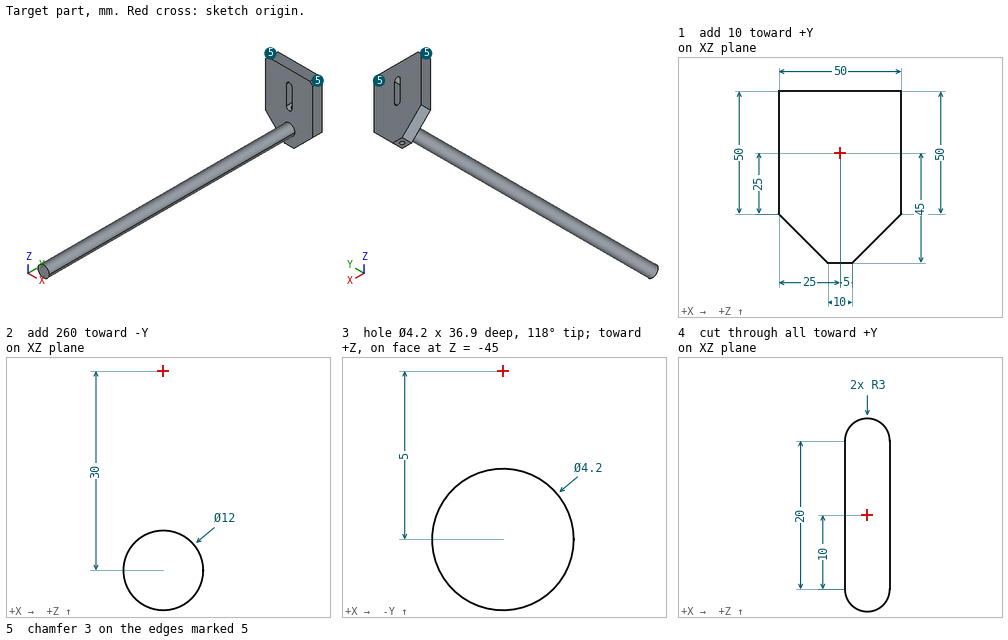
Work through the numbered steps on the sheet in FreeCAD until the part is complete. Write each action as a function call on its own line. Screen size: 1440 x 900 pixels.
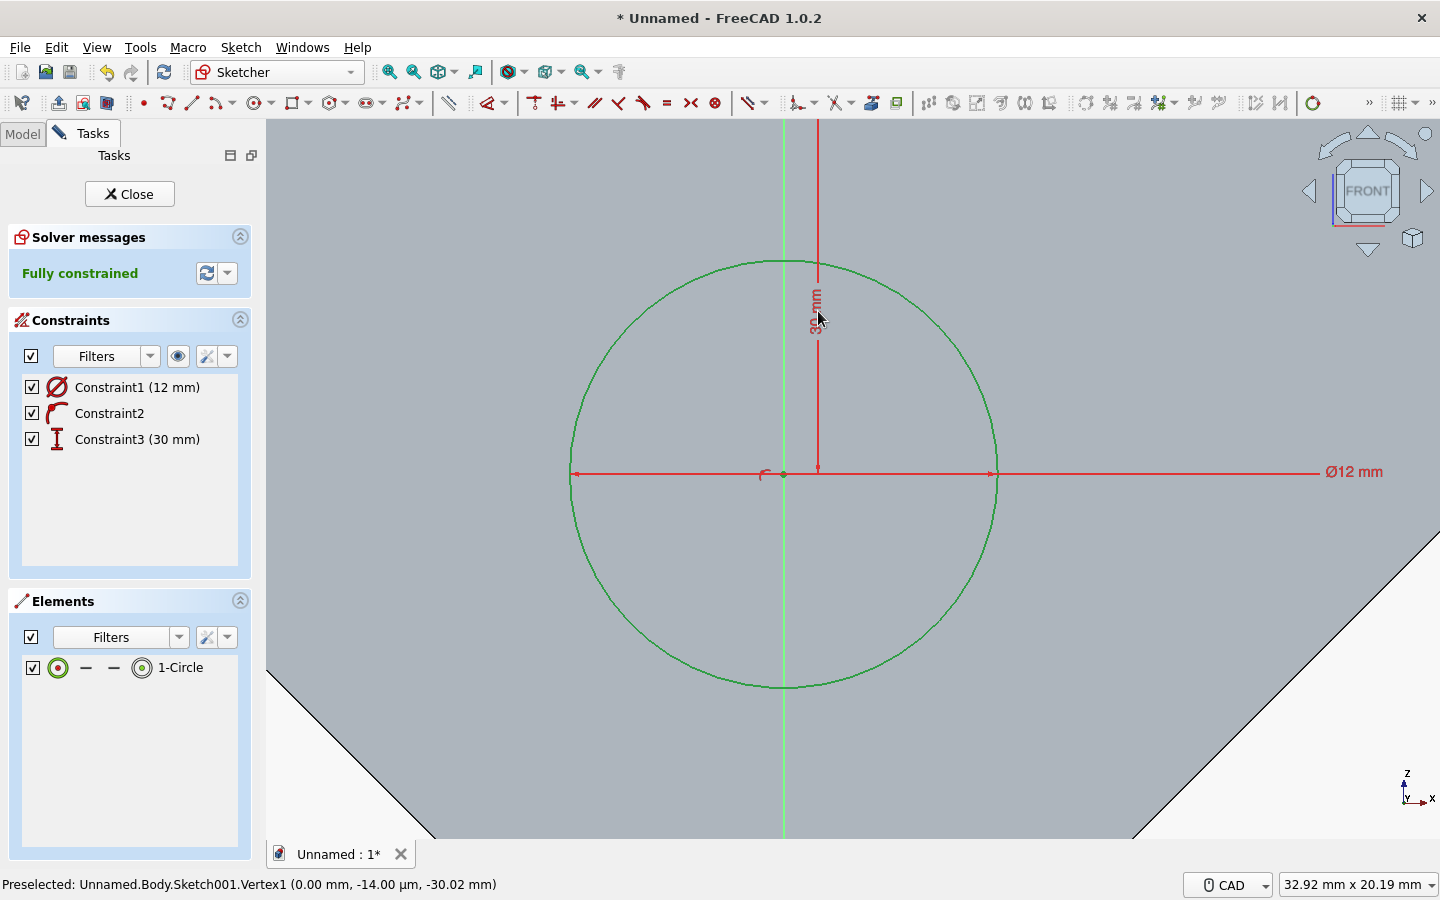
click(130, 194)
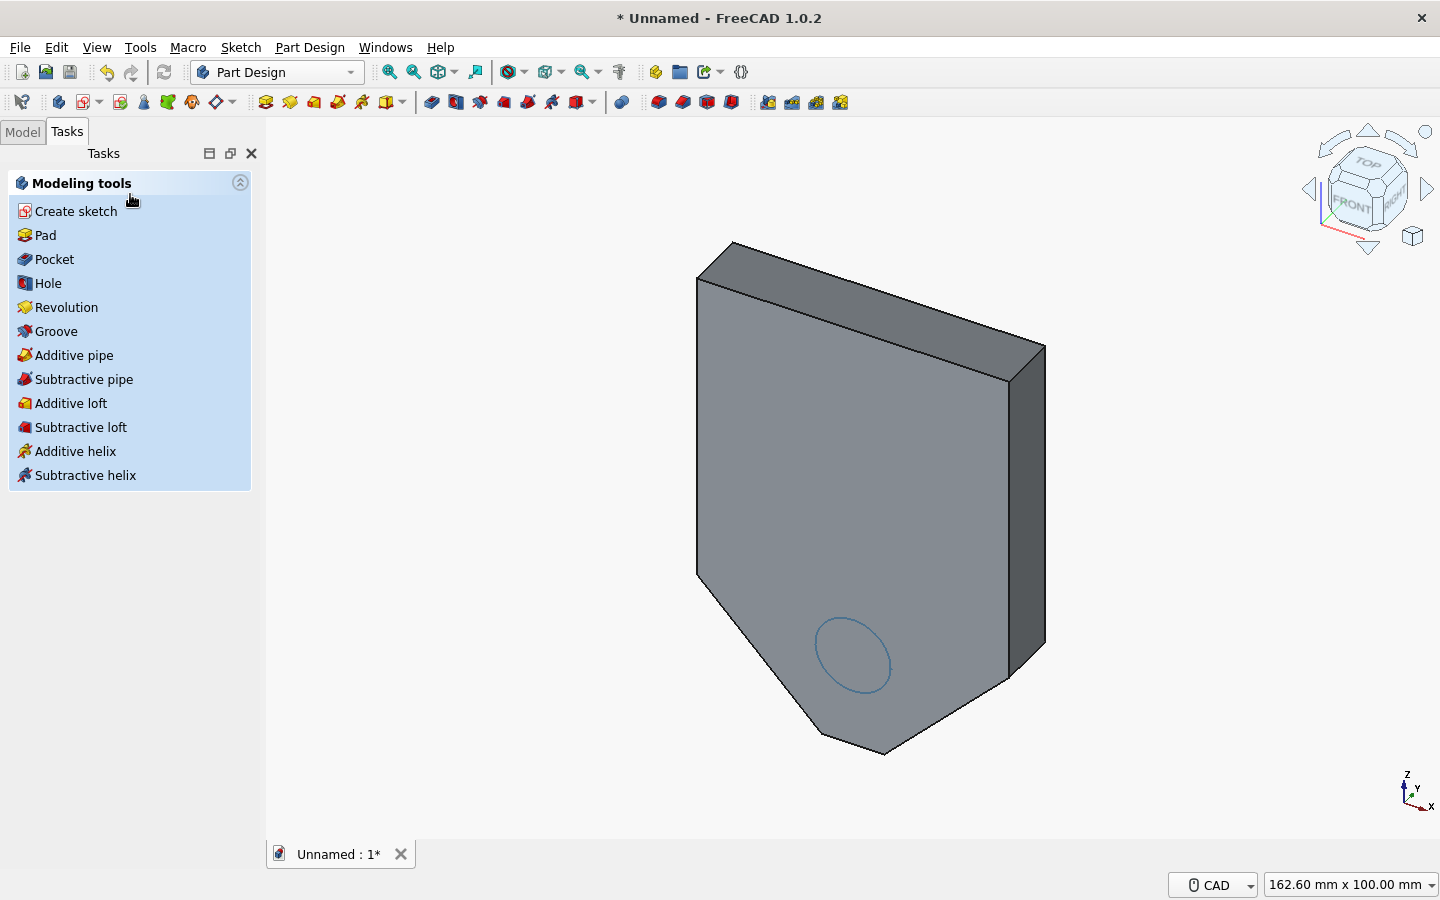
click(266, 102)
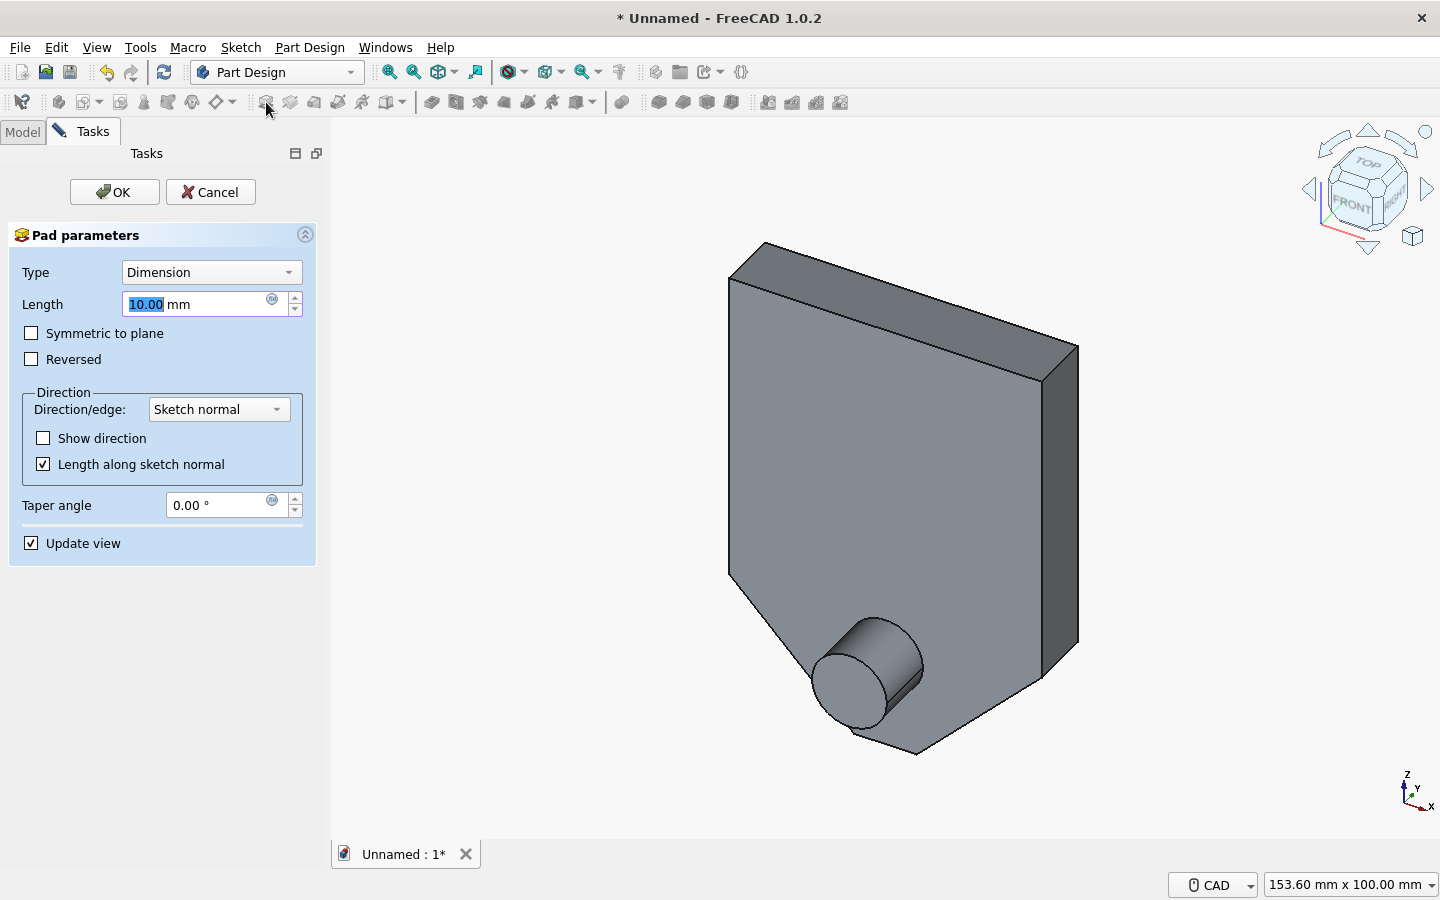
text(260)
key(Tab)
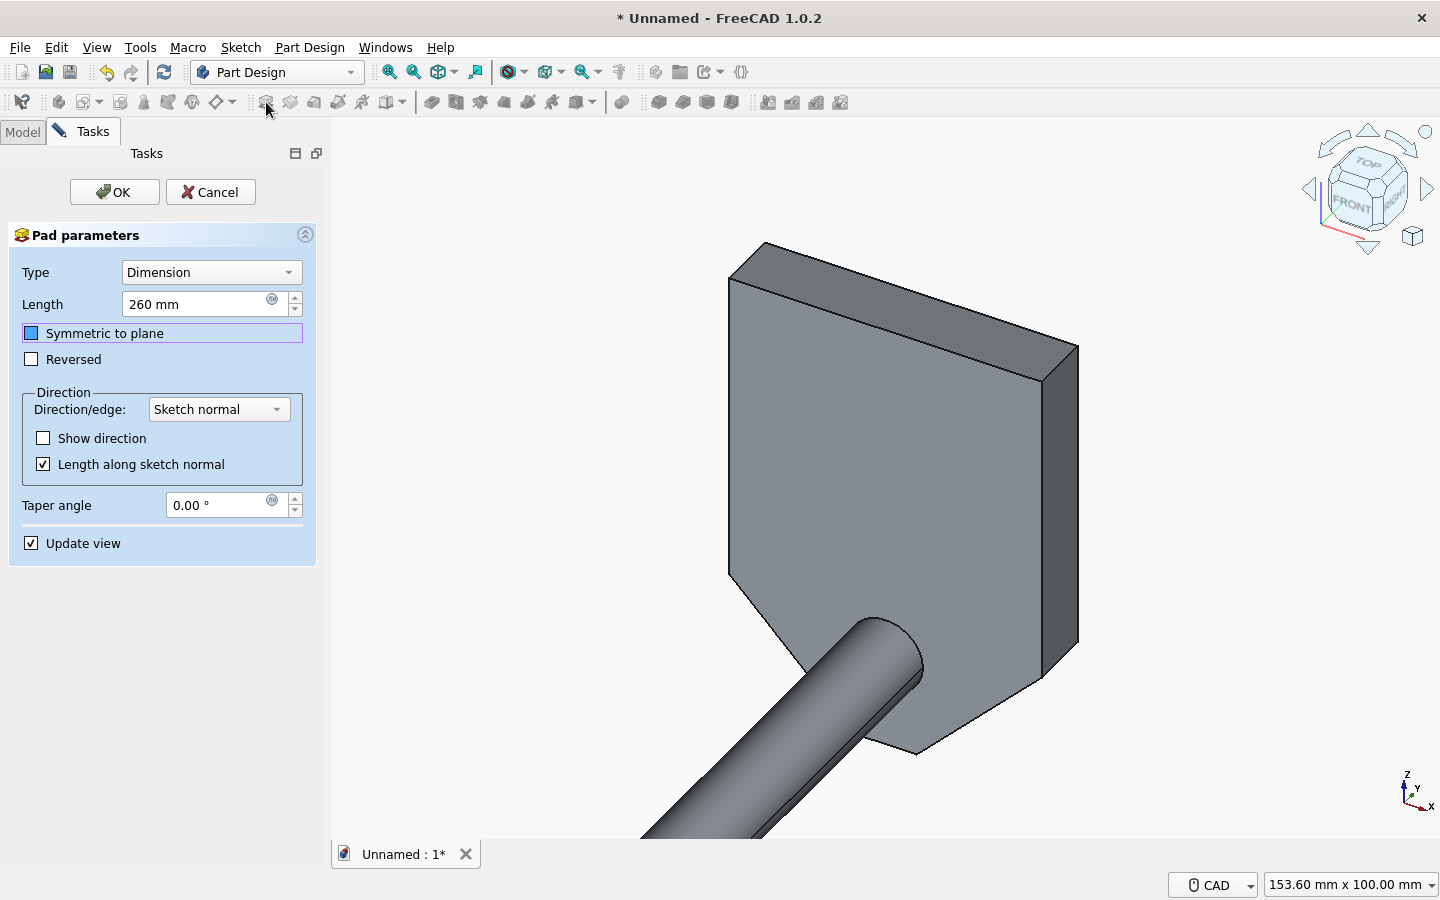
click(115, 192)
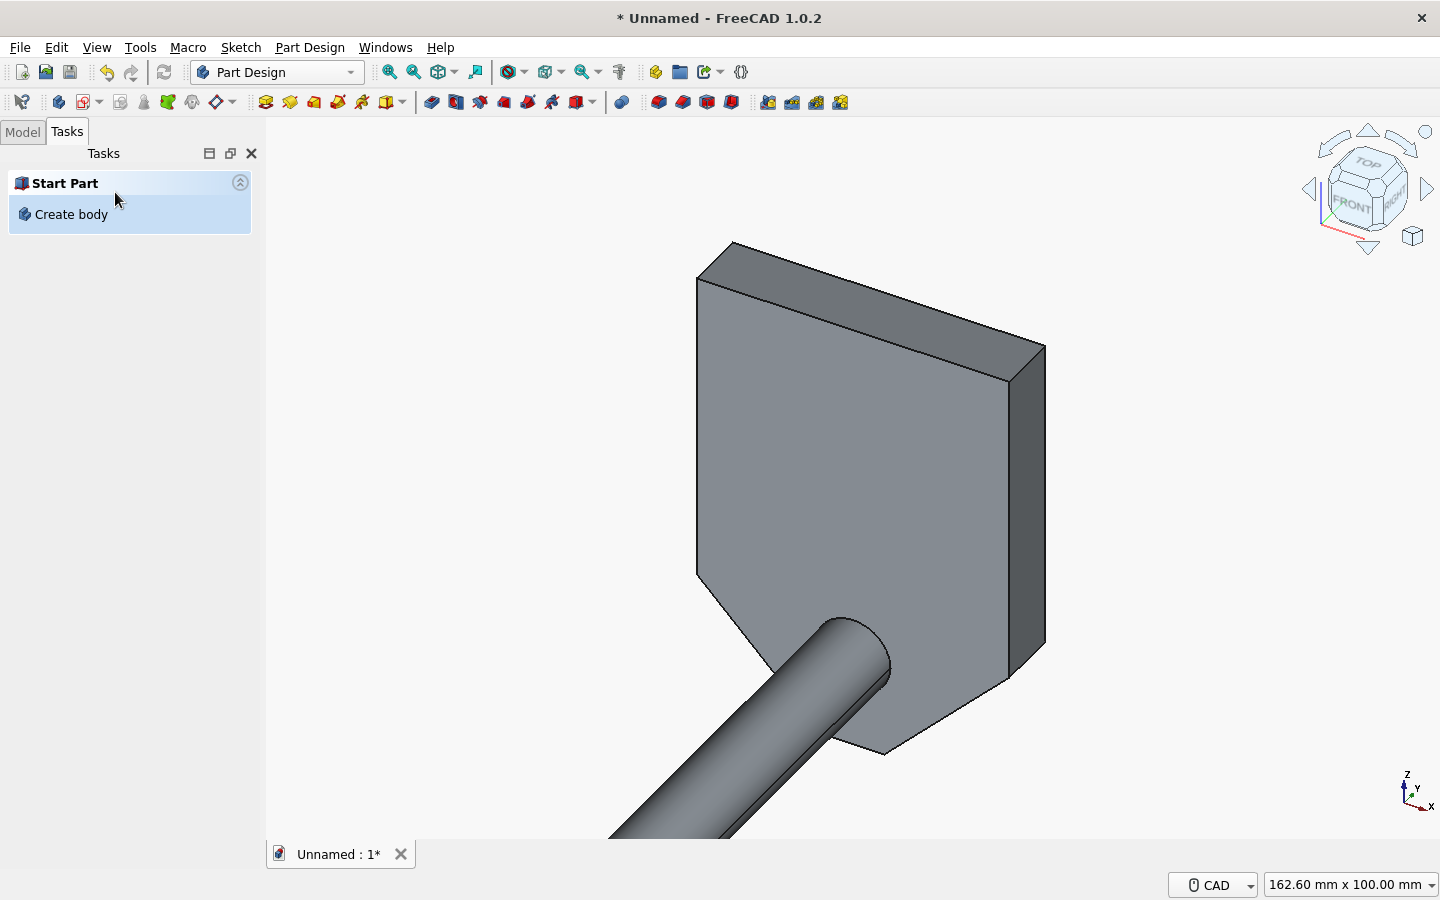
click(390, 72)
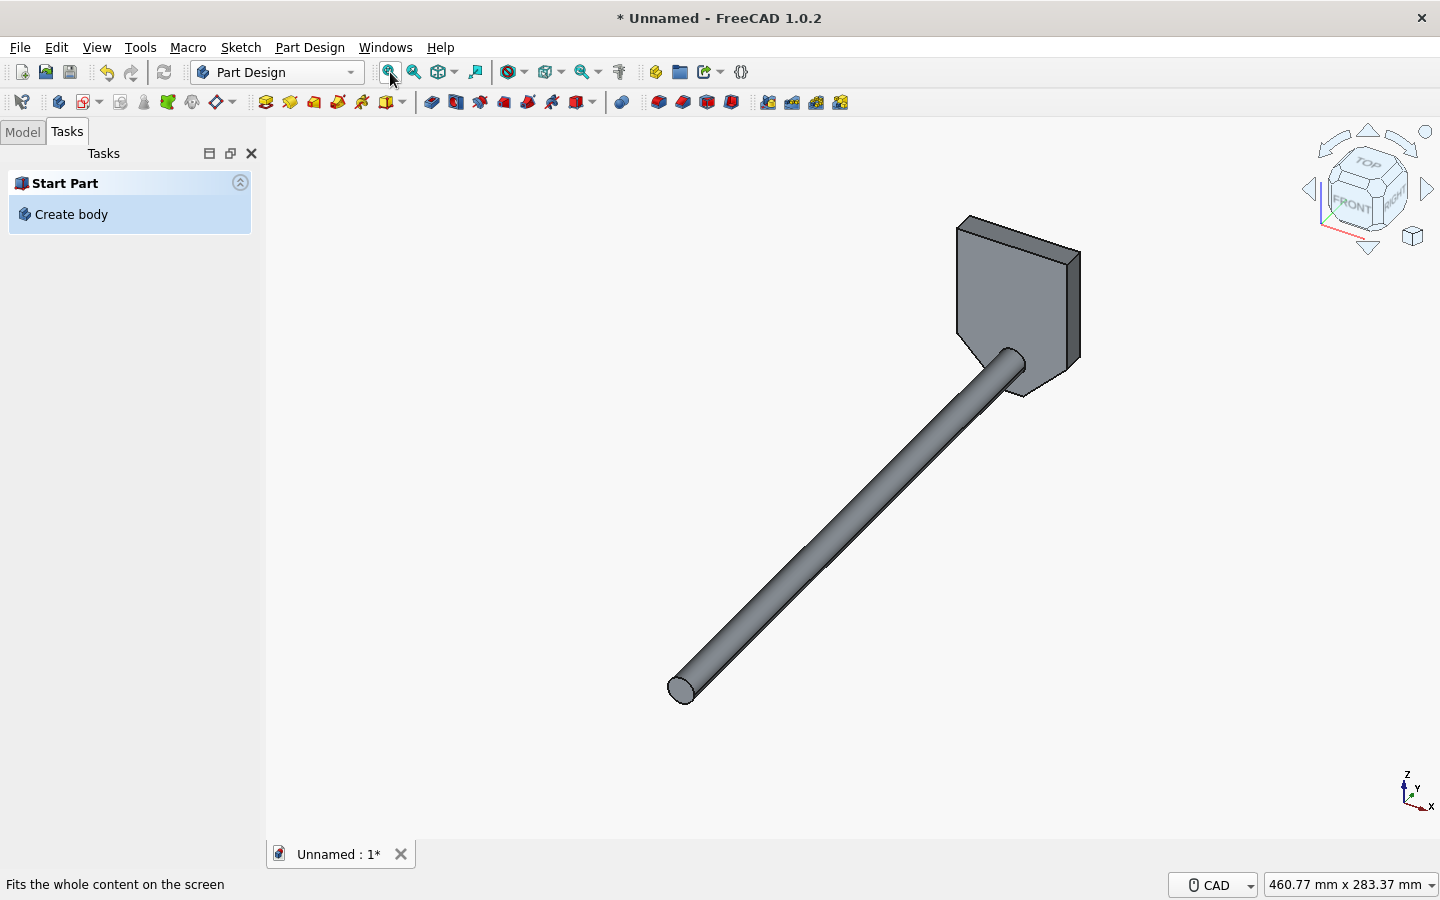
key(5)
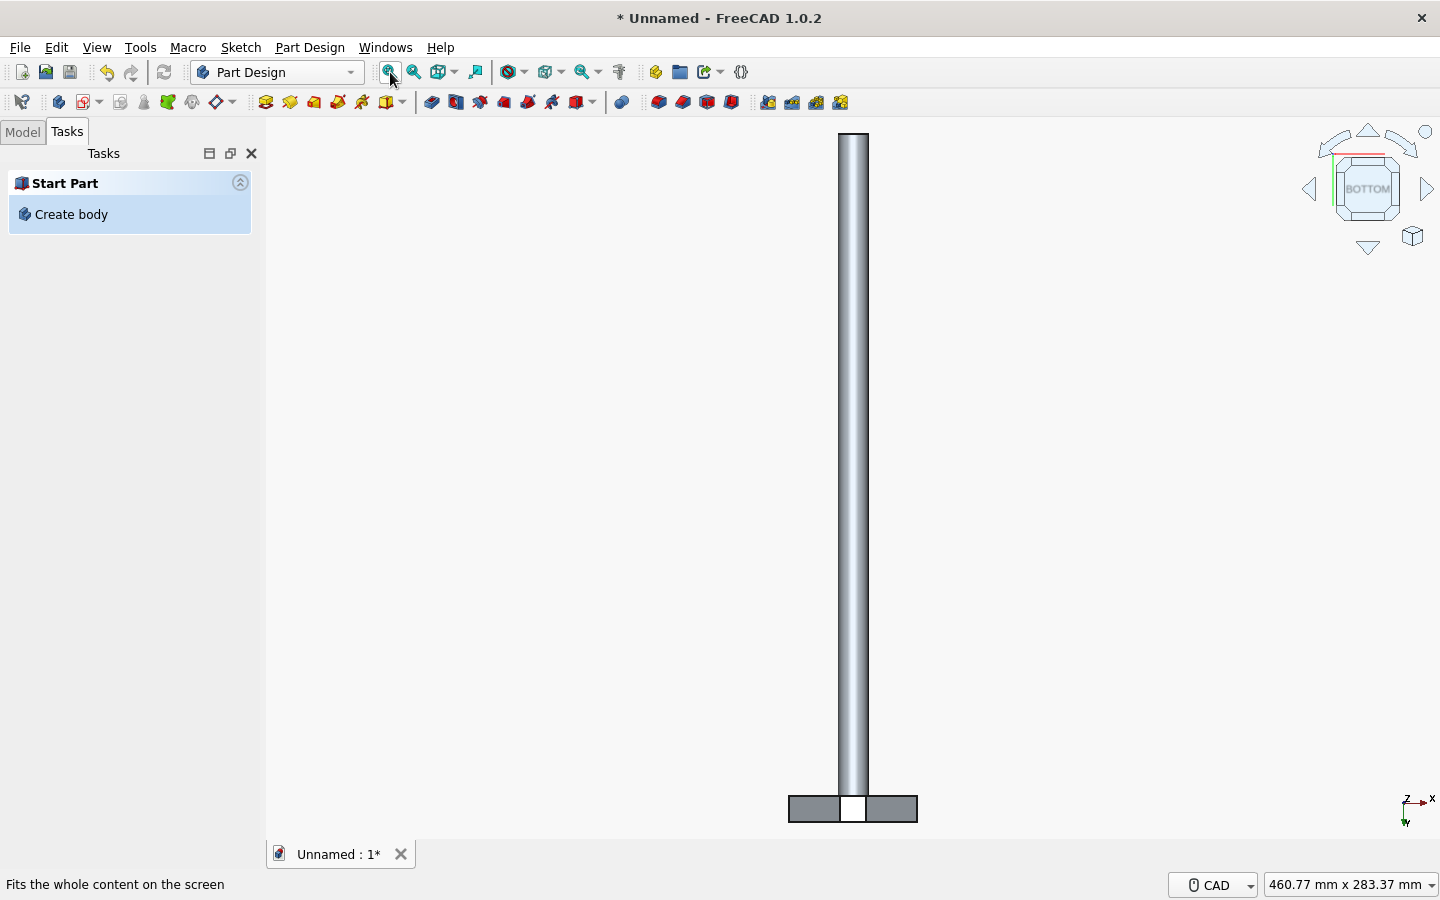
click(853, 808)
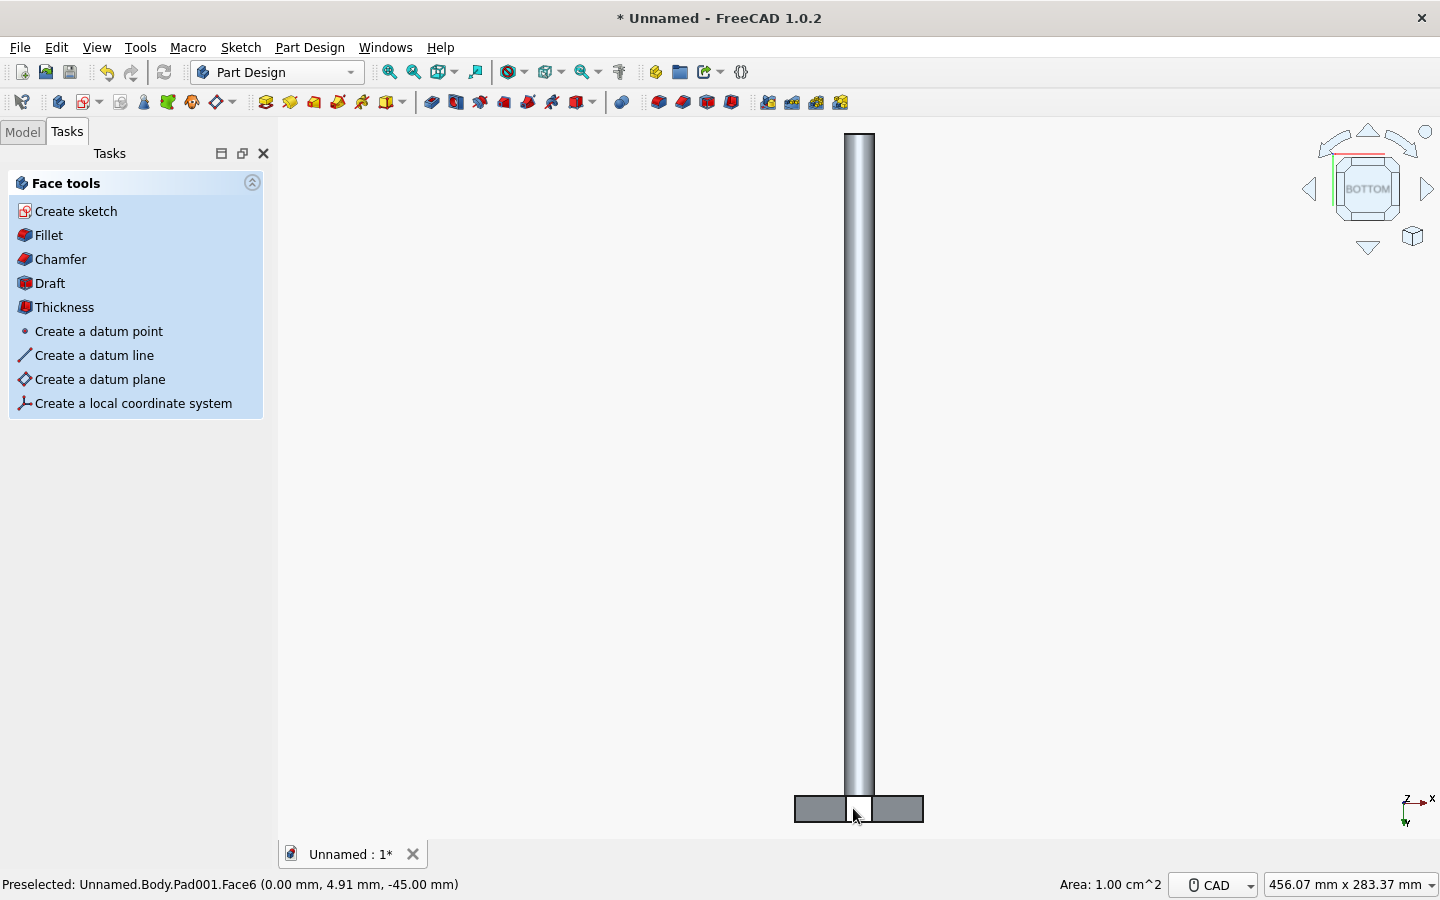
click(84, 102)